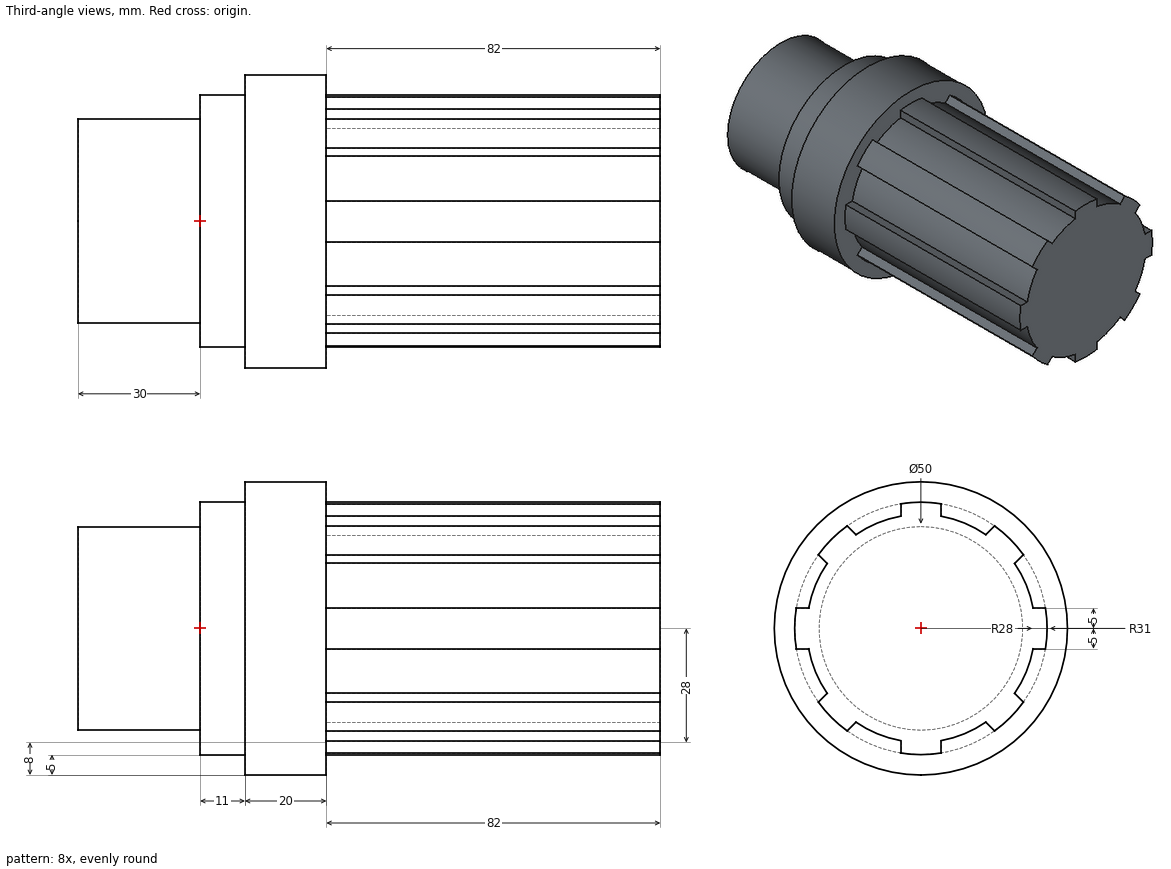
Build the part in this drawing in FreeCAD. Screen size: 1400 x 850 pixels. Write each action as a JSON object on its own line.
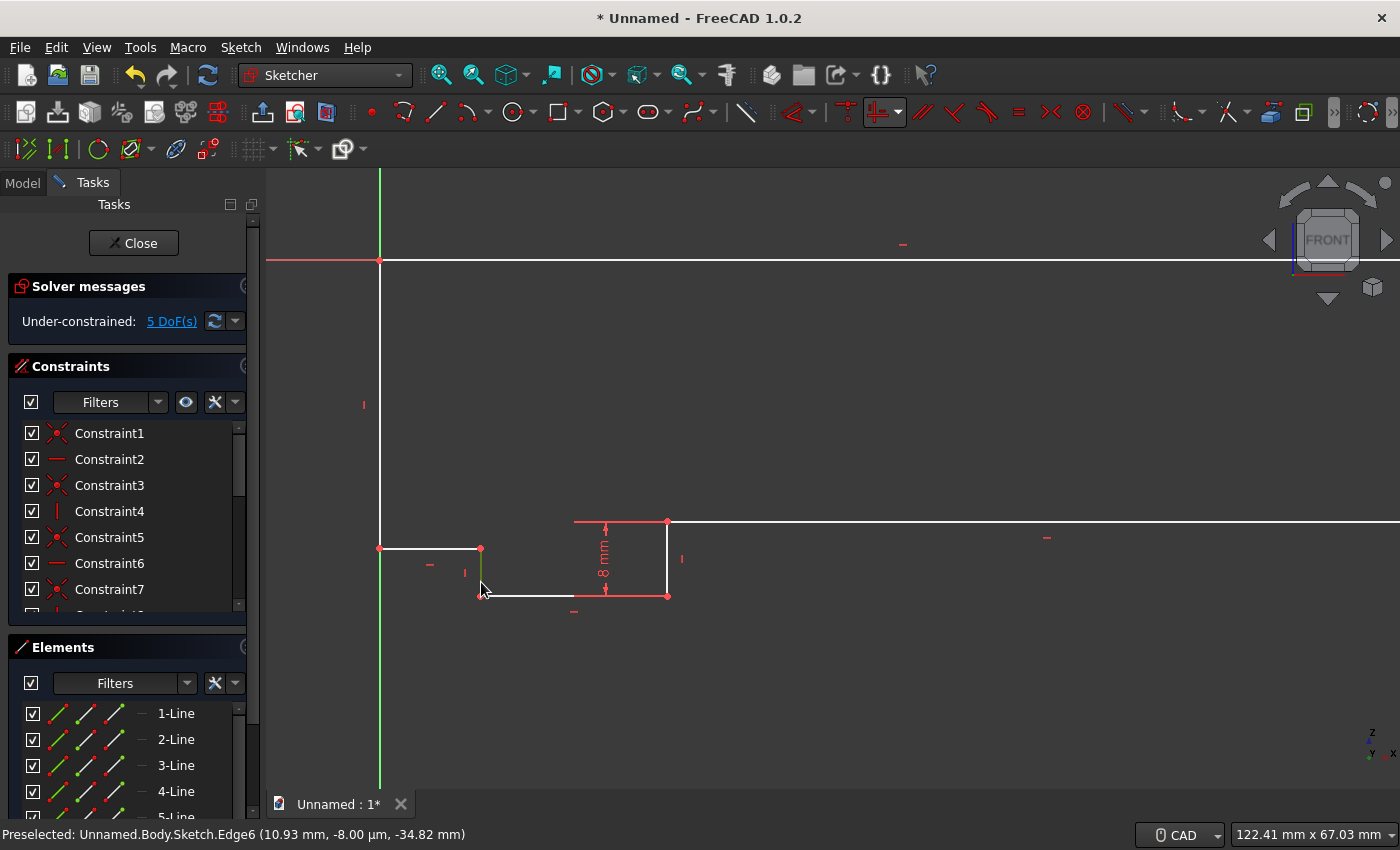
{"action": "key", "text": "i"}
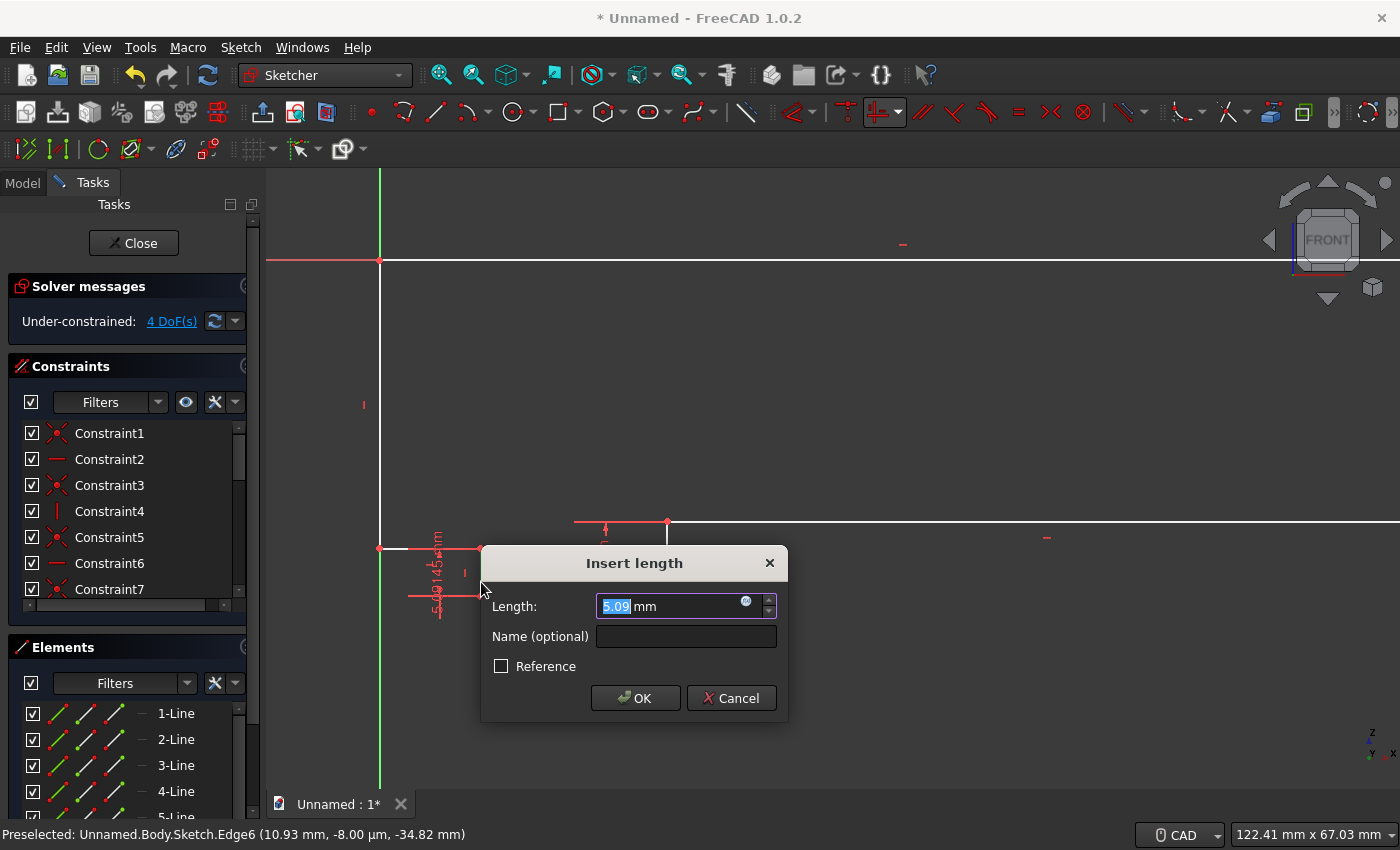
{"action": "type", "text": "5"}
{"action": "key", "text": "Return"}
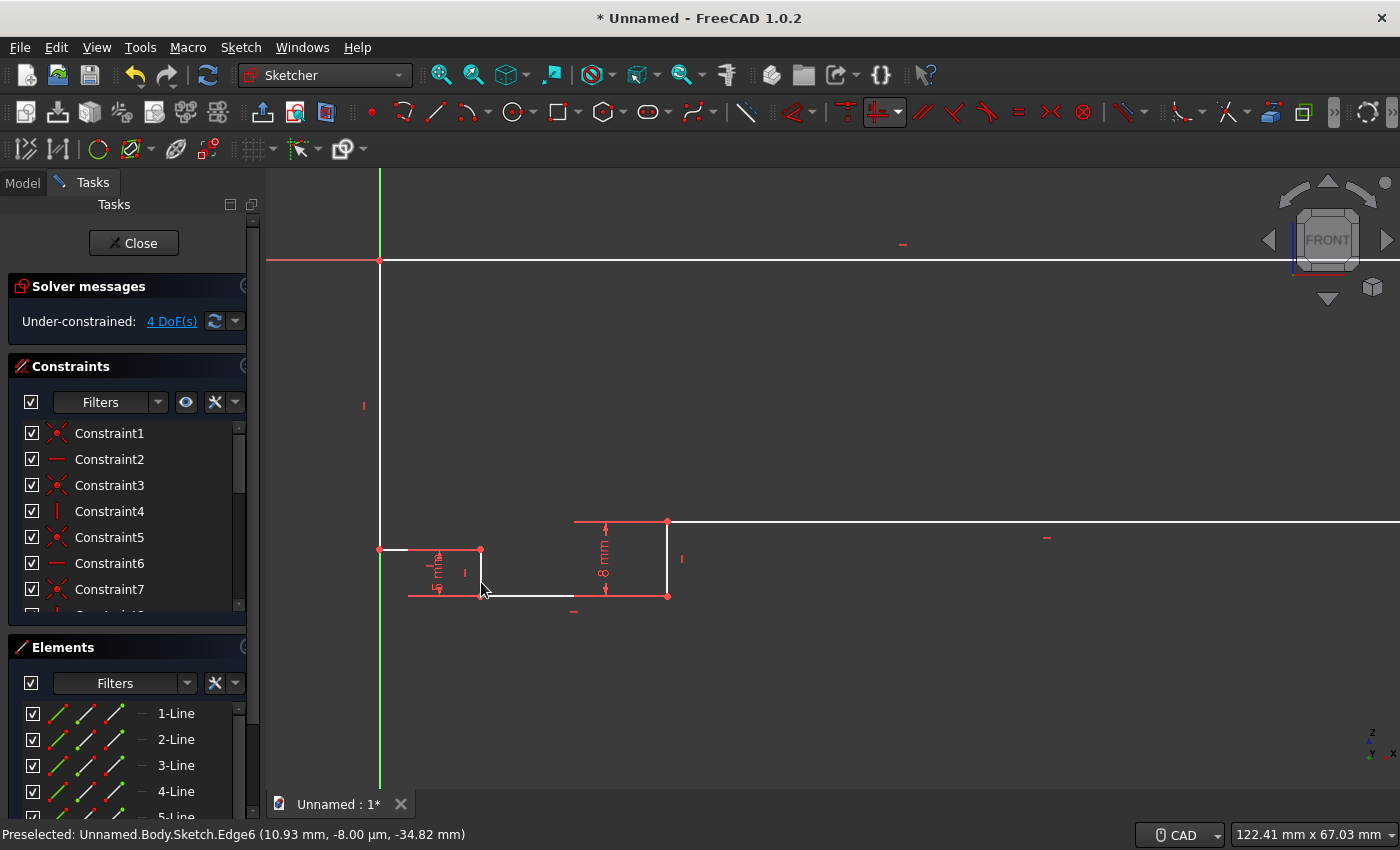
{"action": "scroll", "coordinate": [483, 583], "scroll_direction": "down", "scroll_amount": 2}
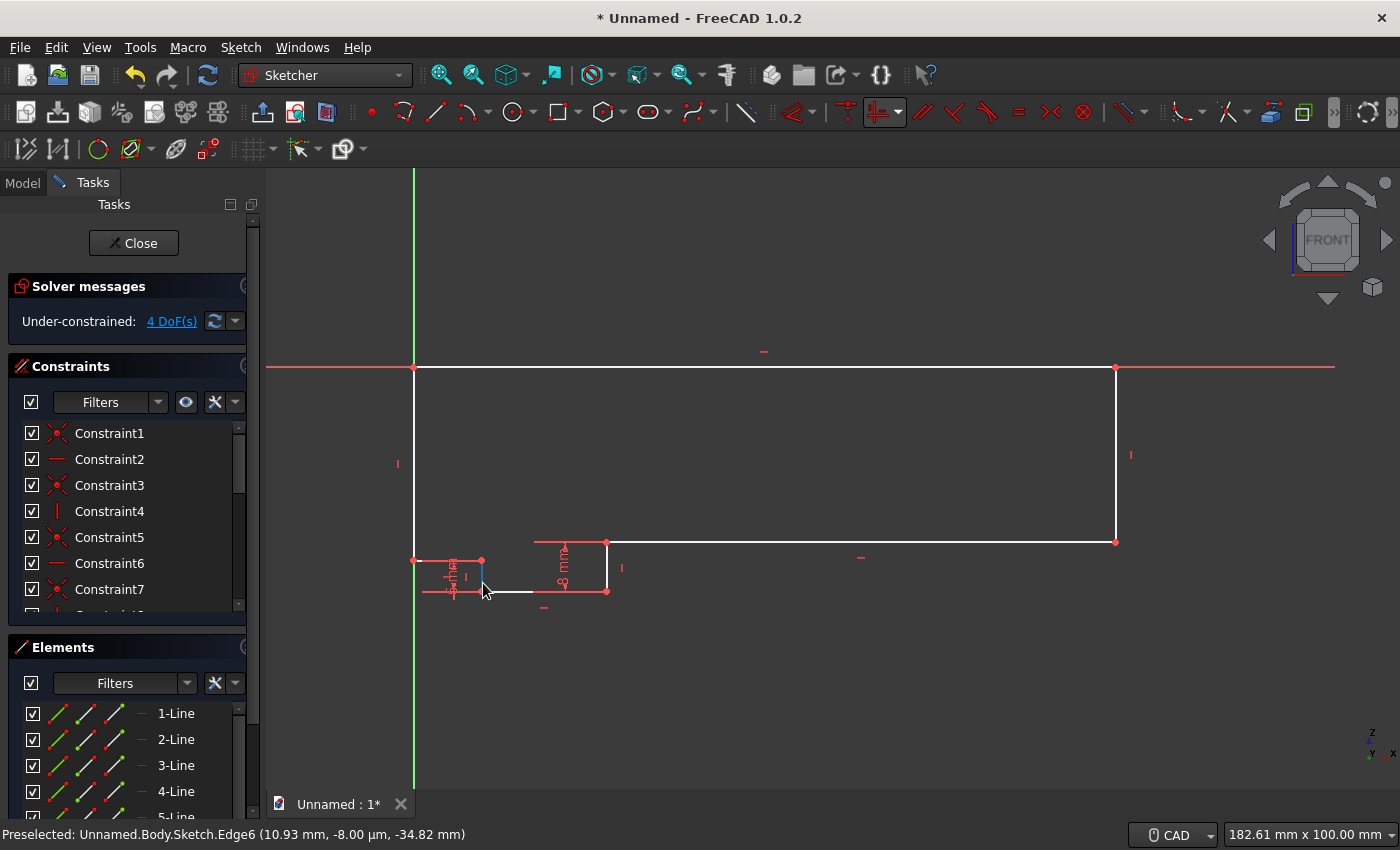
{"action": "left_click", "coordinate": [1116, 420]}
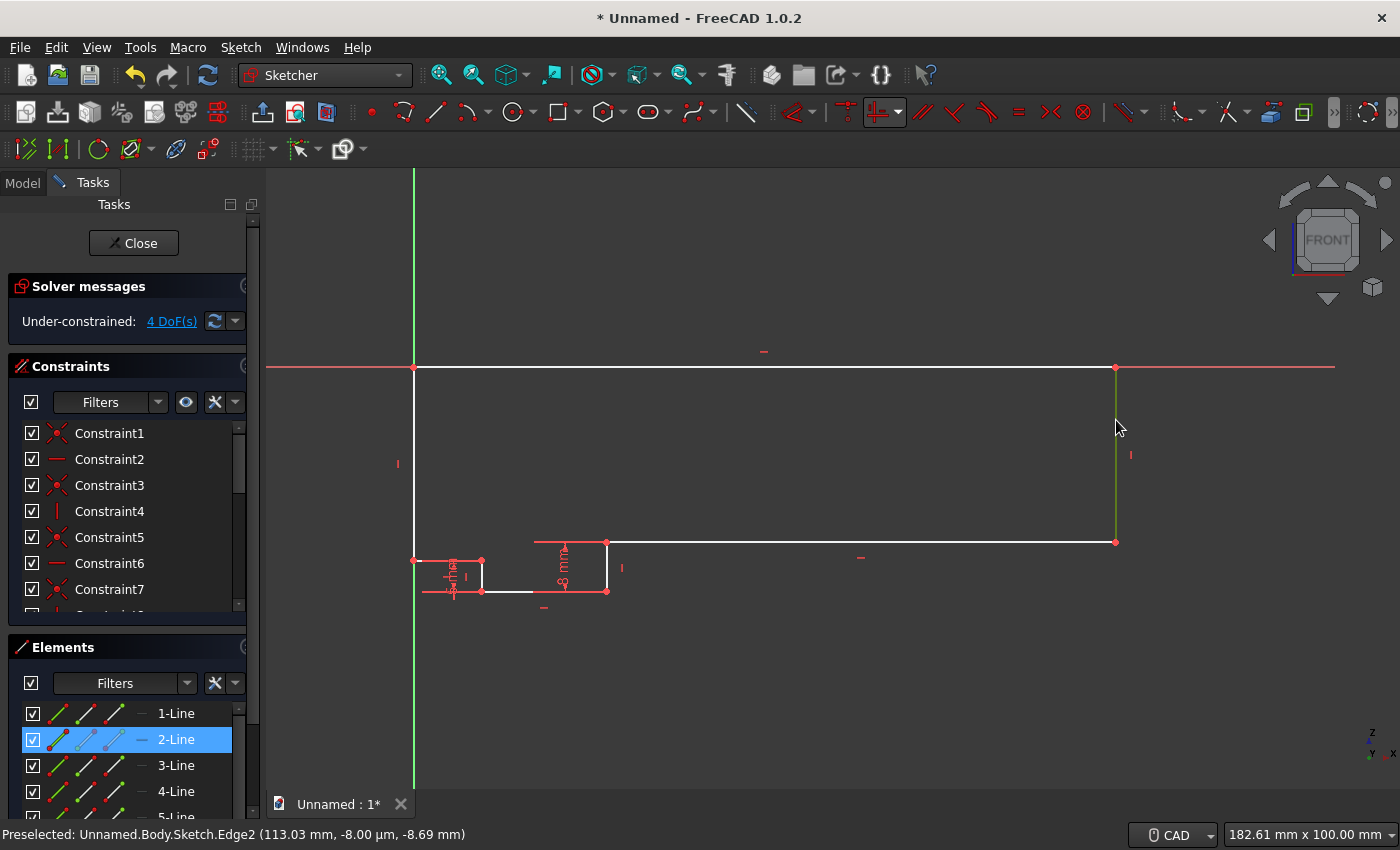
{"action": "key", "text": "i"}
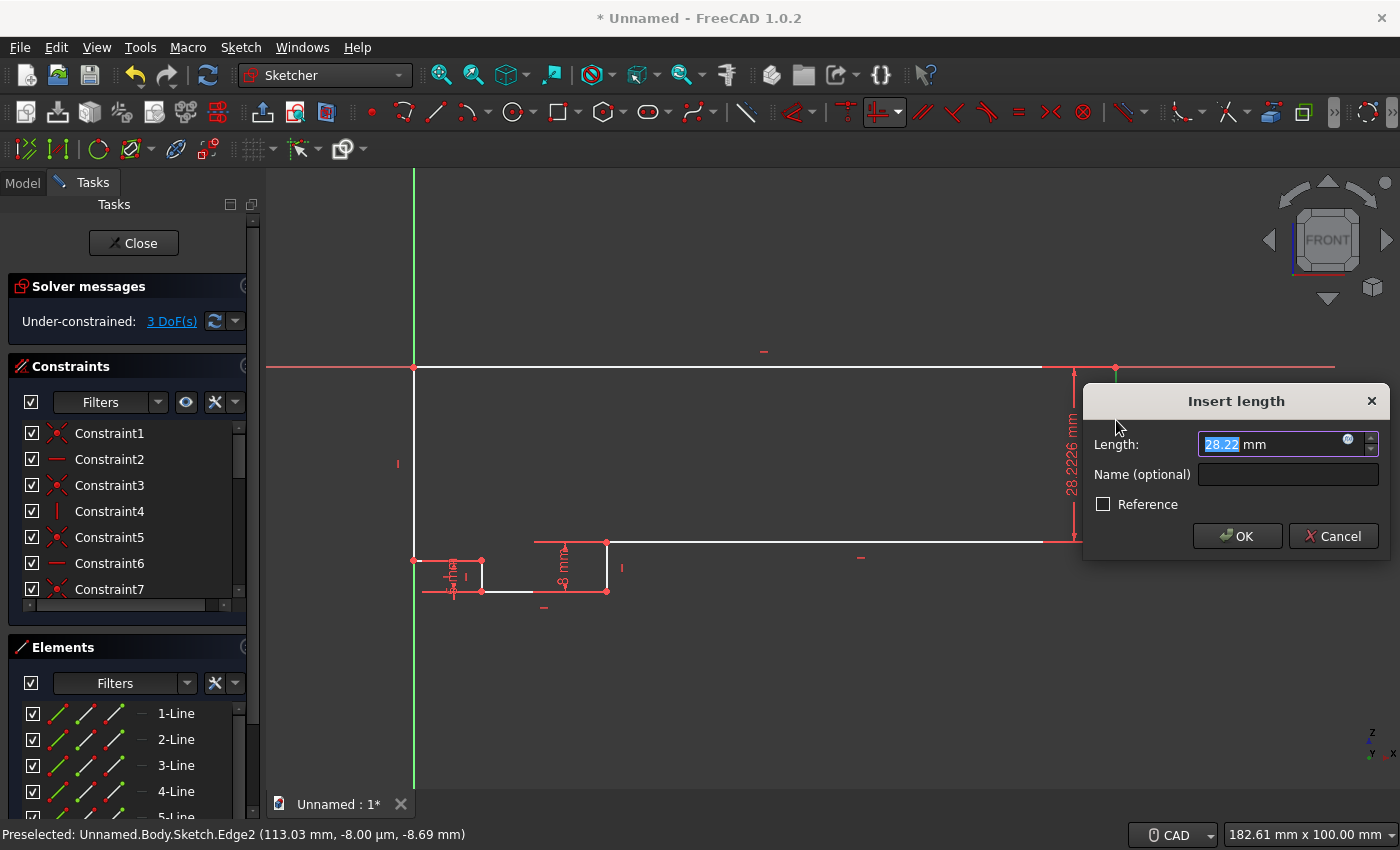
{"action": "type", "text": "28"}
{"action": "key", "text": "Return"}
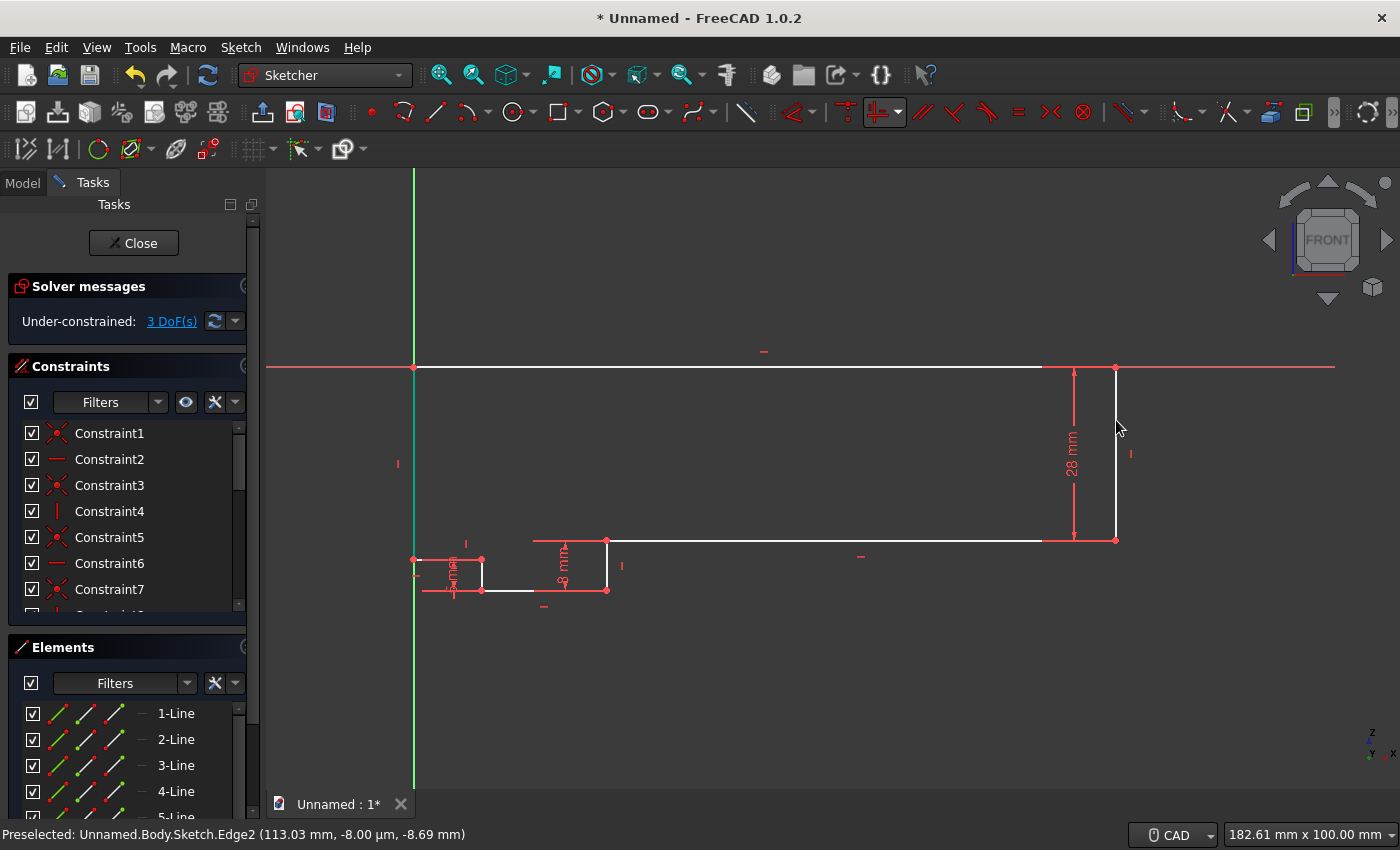
{"action": "left_click", "coordinate": [963, 541]}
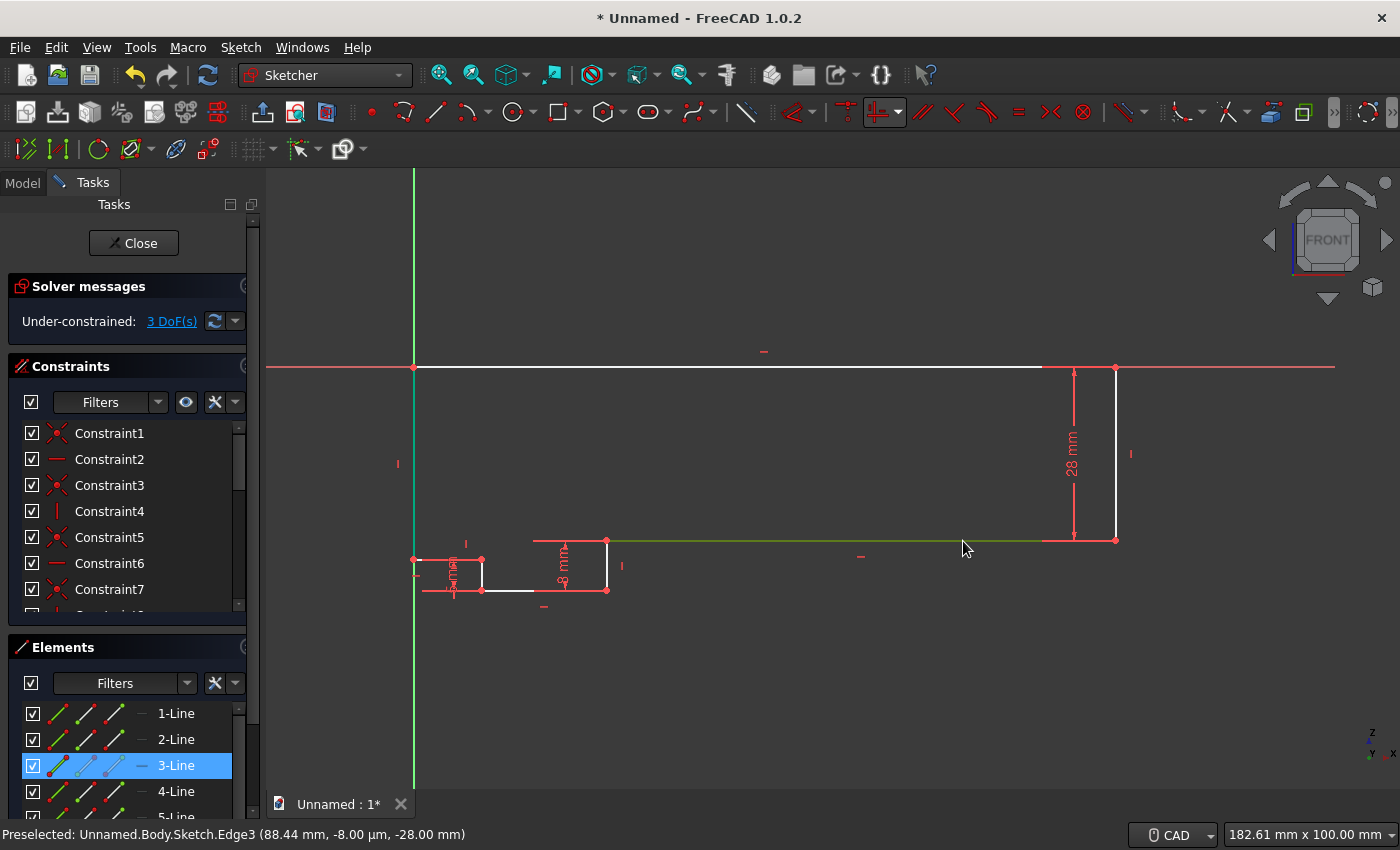
{"action": "left_click", "coordinate": [814, 112]}